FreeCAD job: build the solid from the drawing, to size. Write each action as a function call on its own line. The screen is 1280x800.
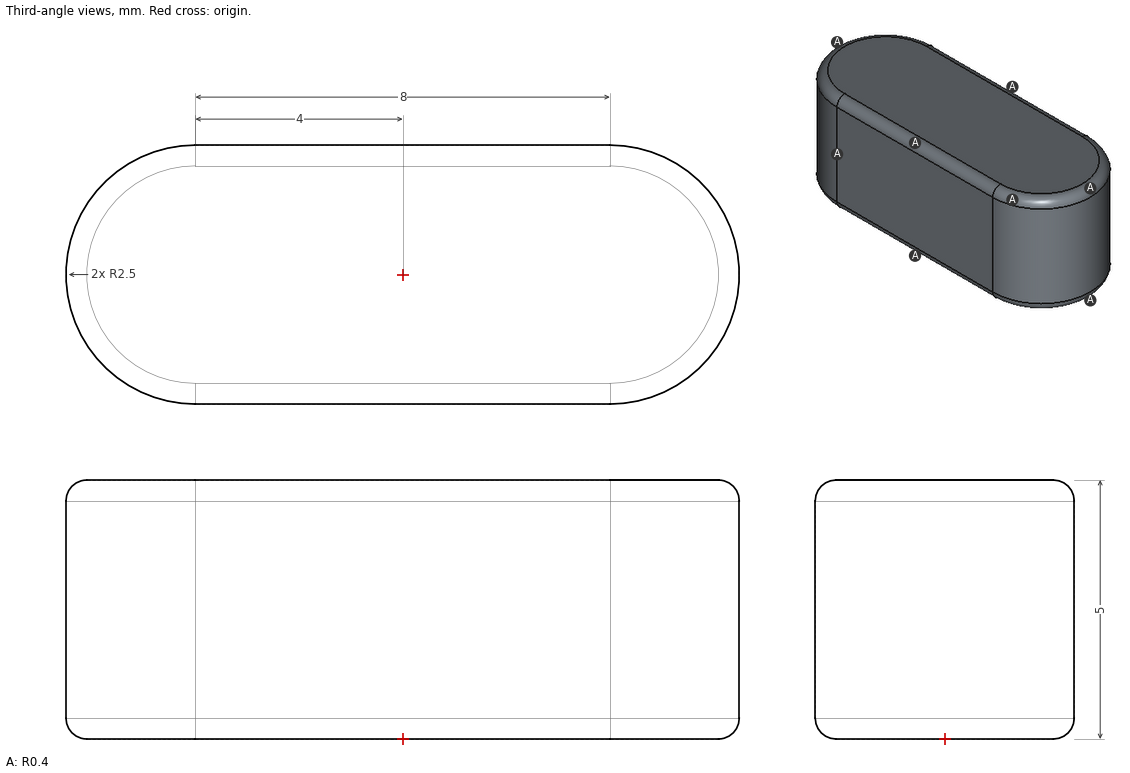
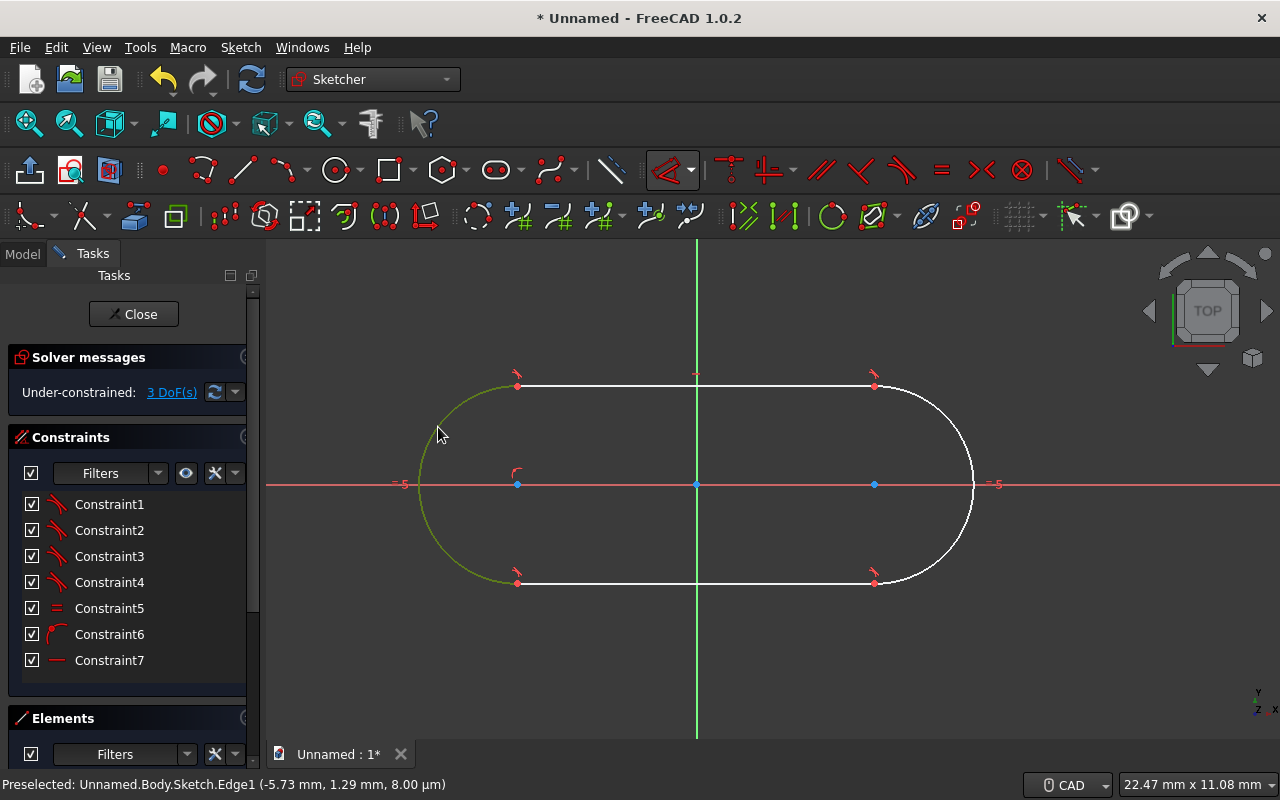
key(k)
key(r)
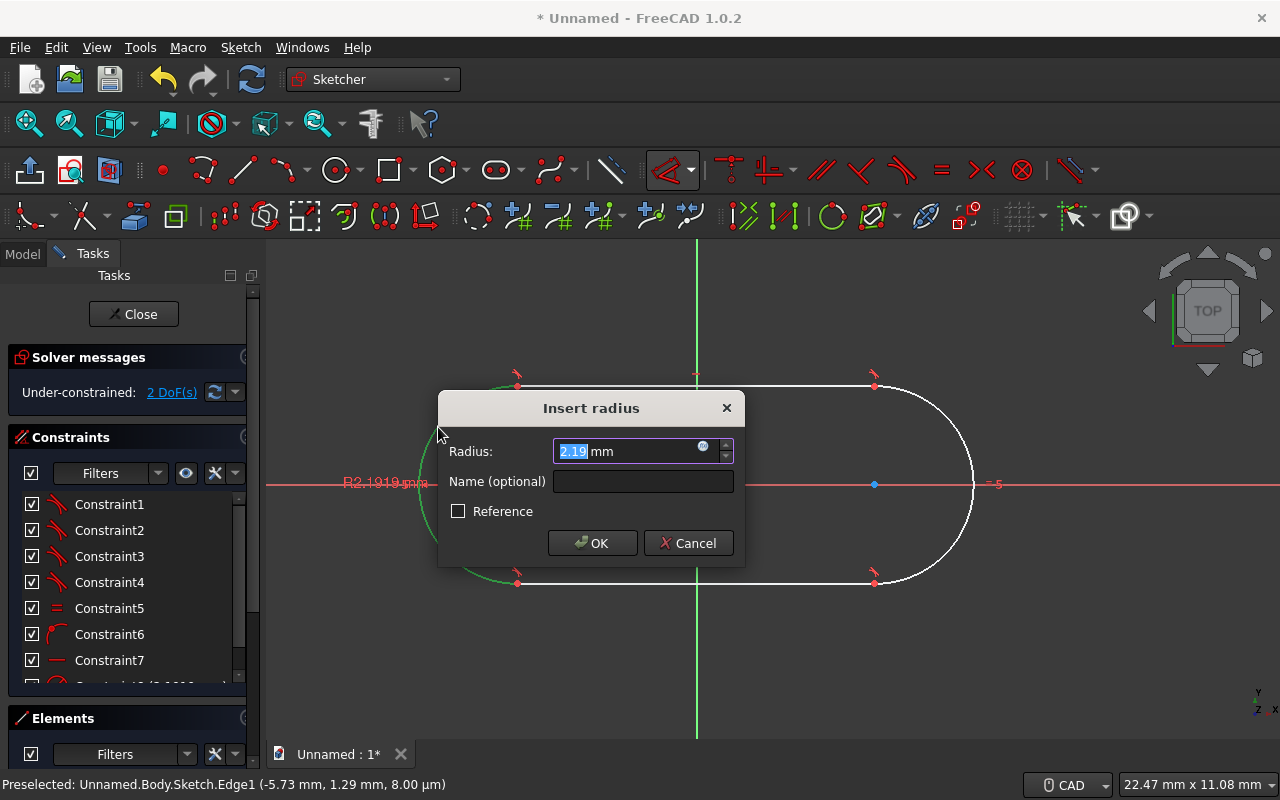
text(2.5)
key(Return)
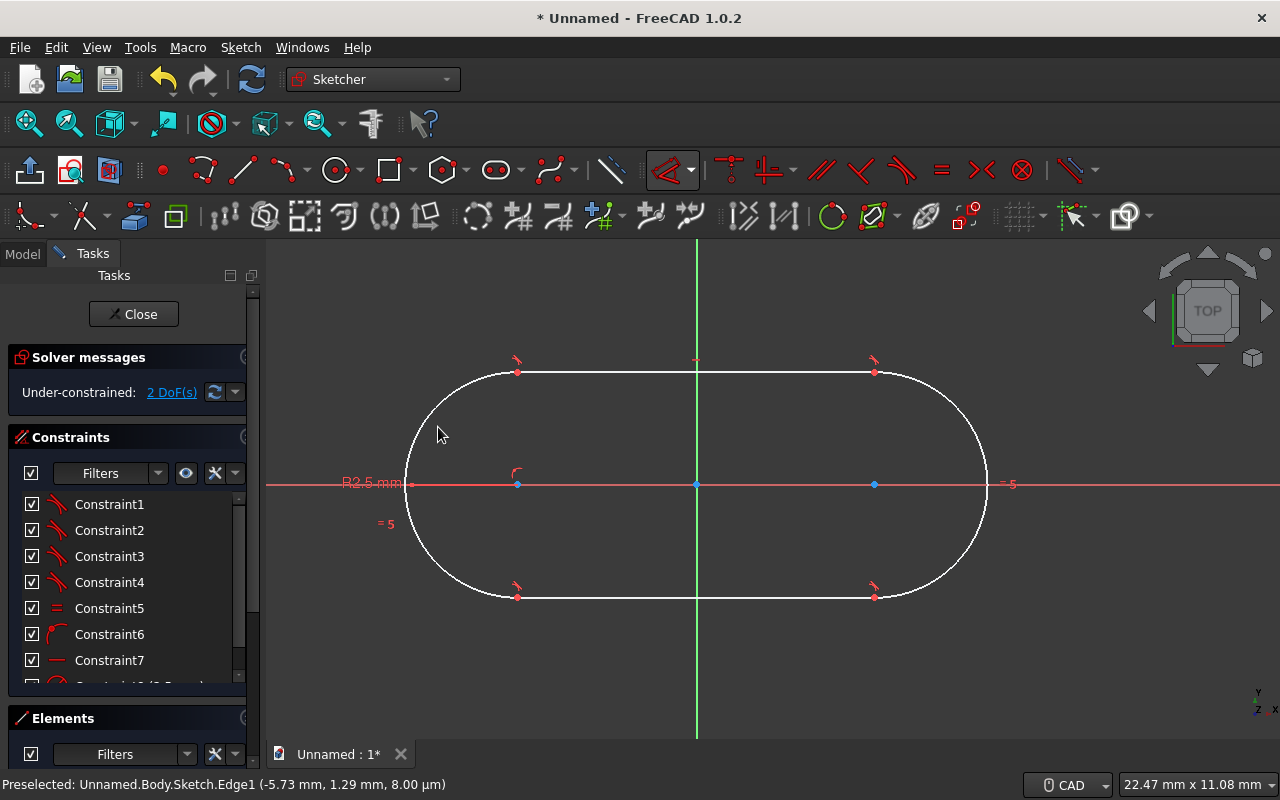
click(625, 372)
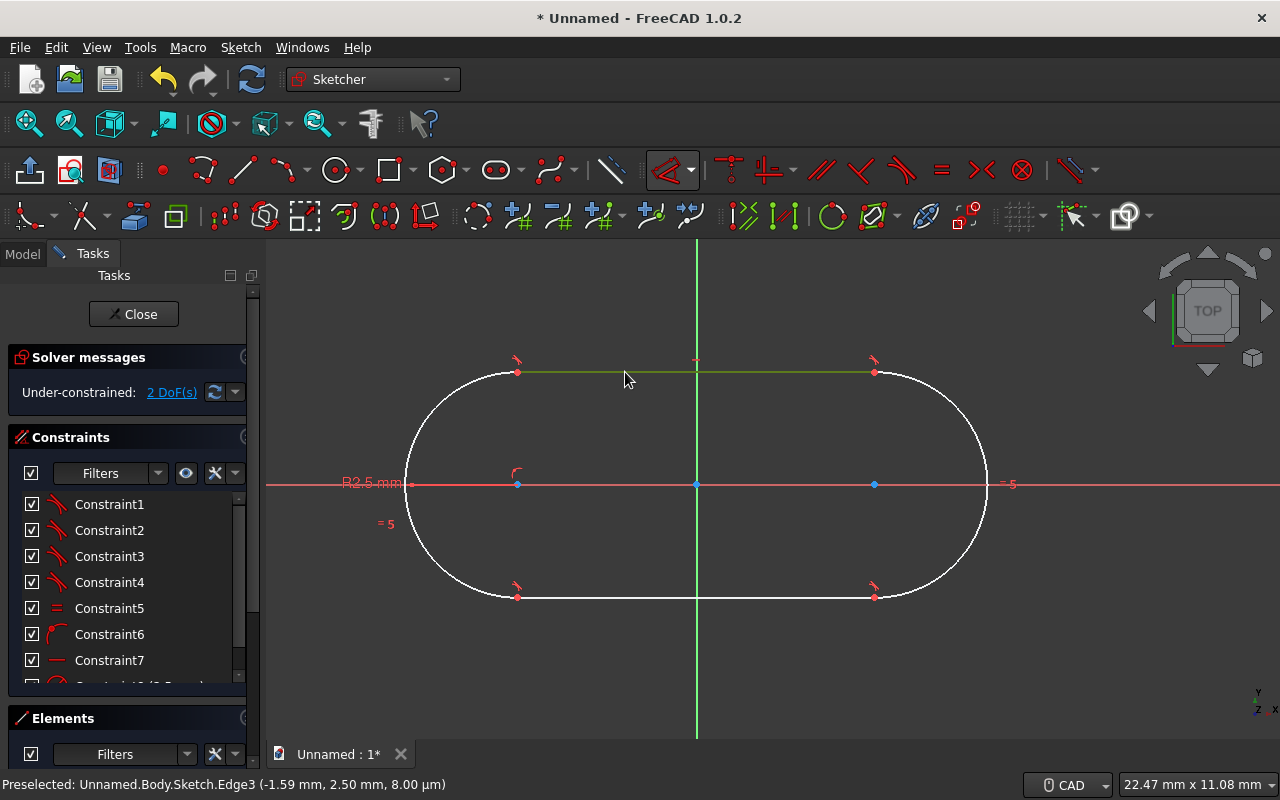
key(l)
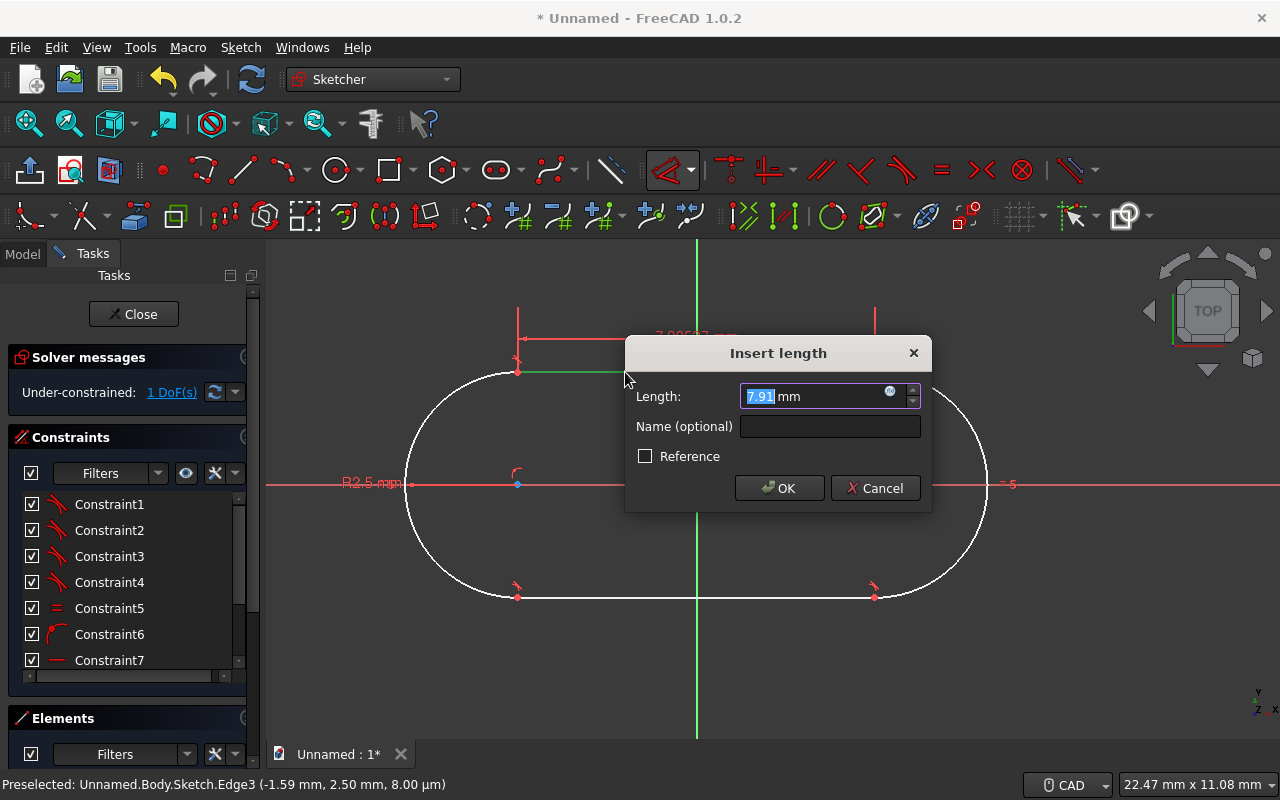
text(8)
key(Return)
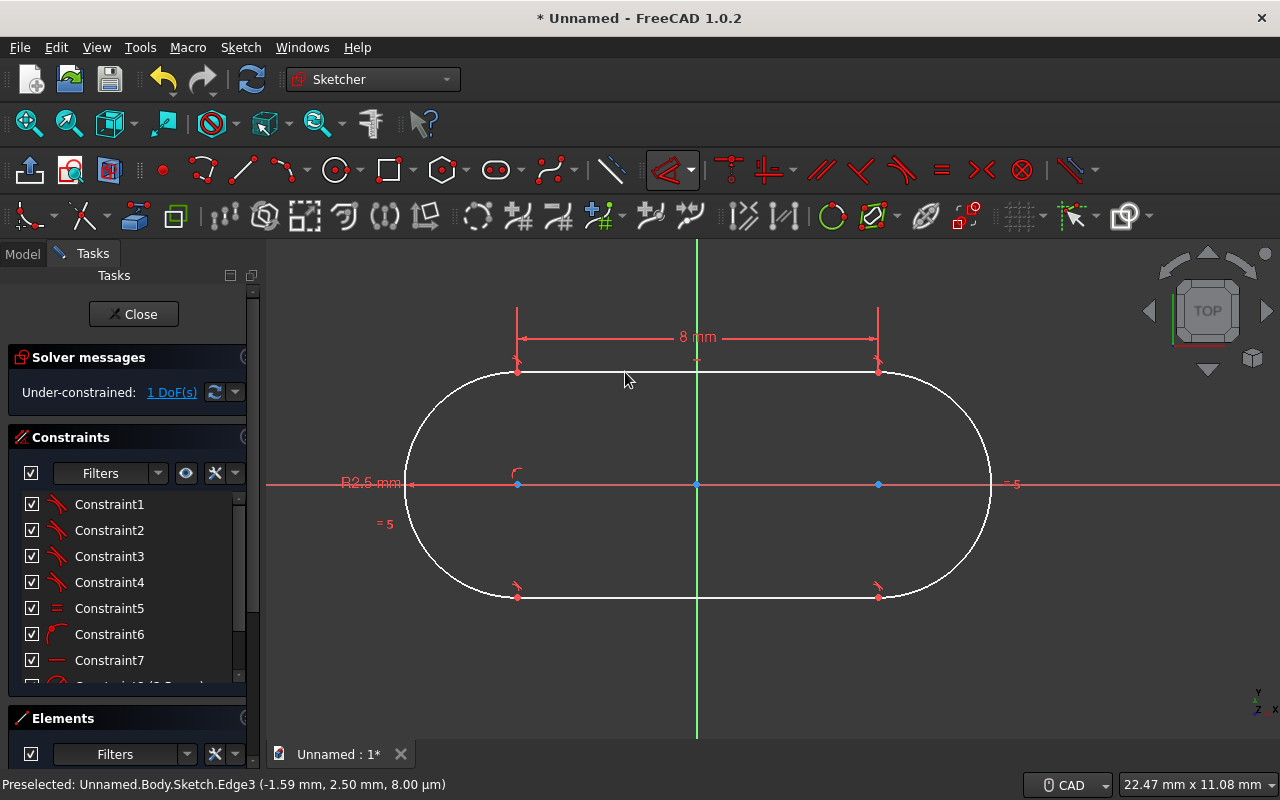
click(517, 372)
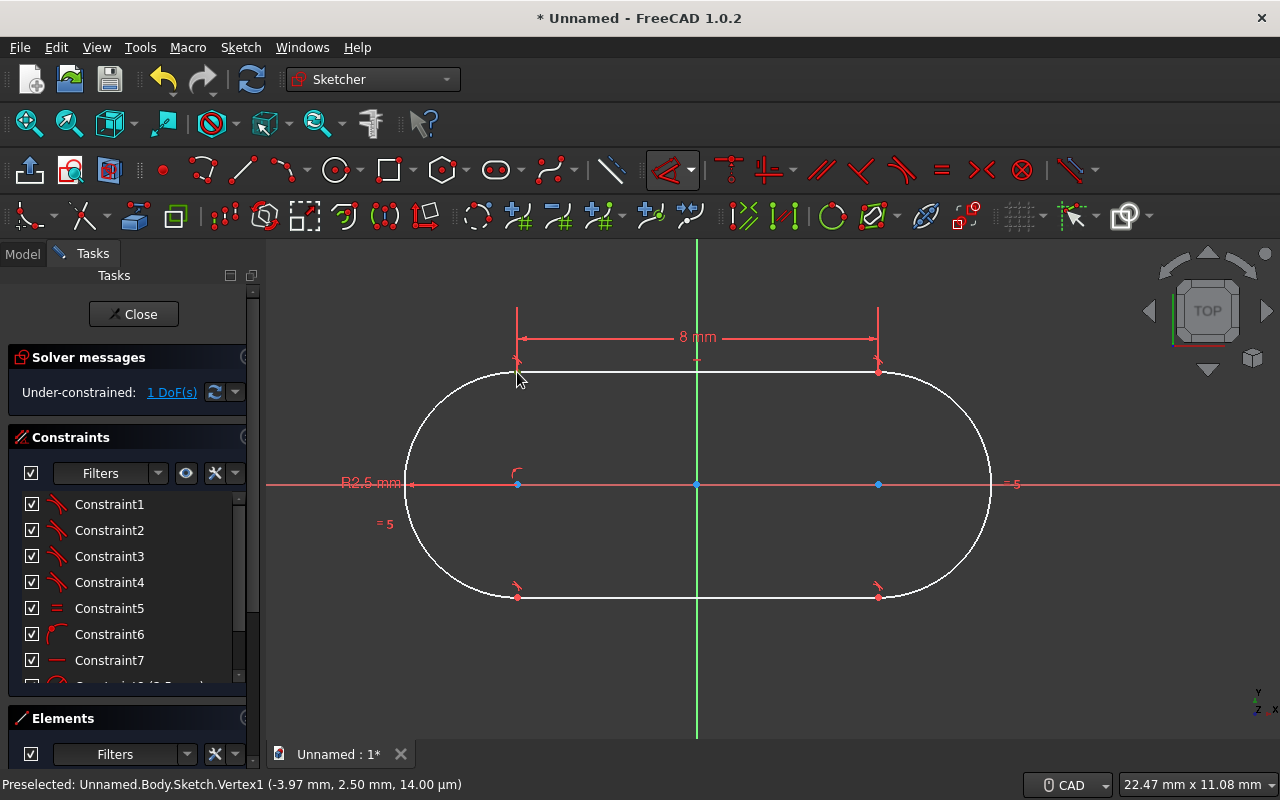
click(694, 170)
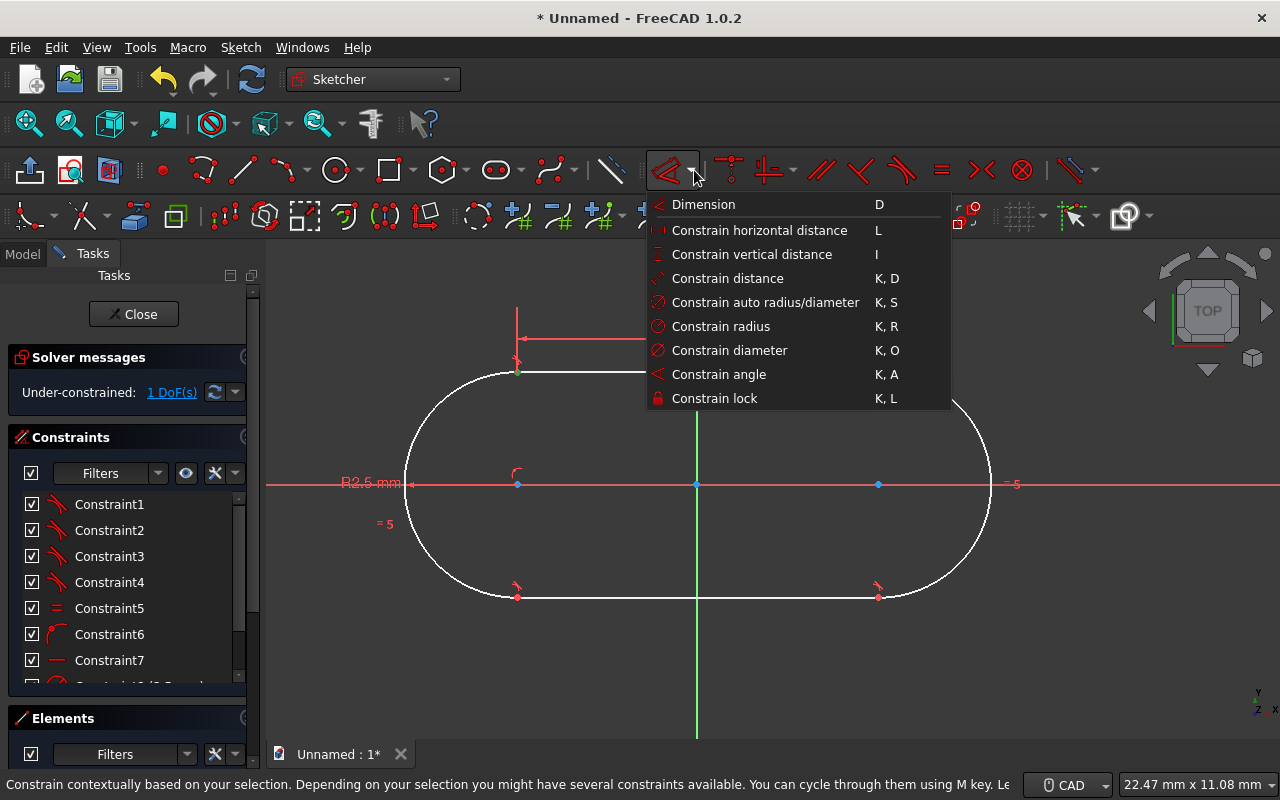
click(799, 230)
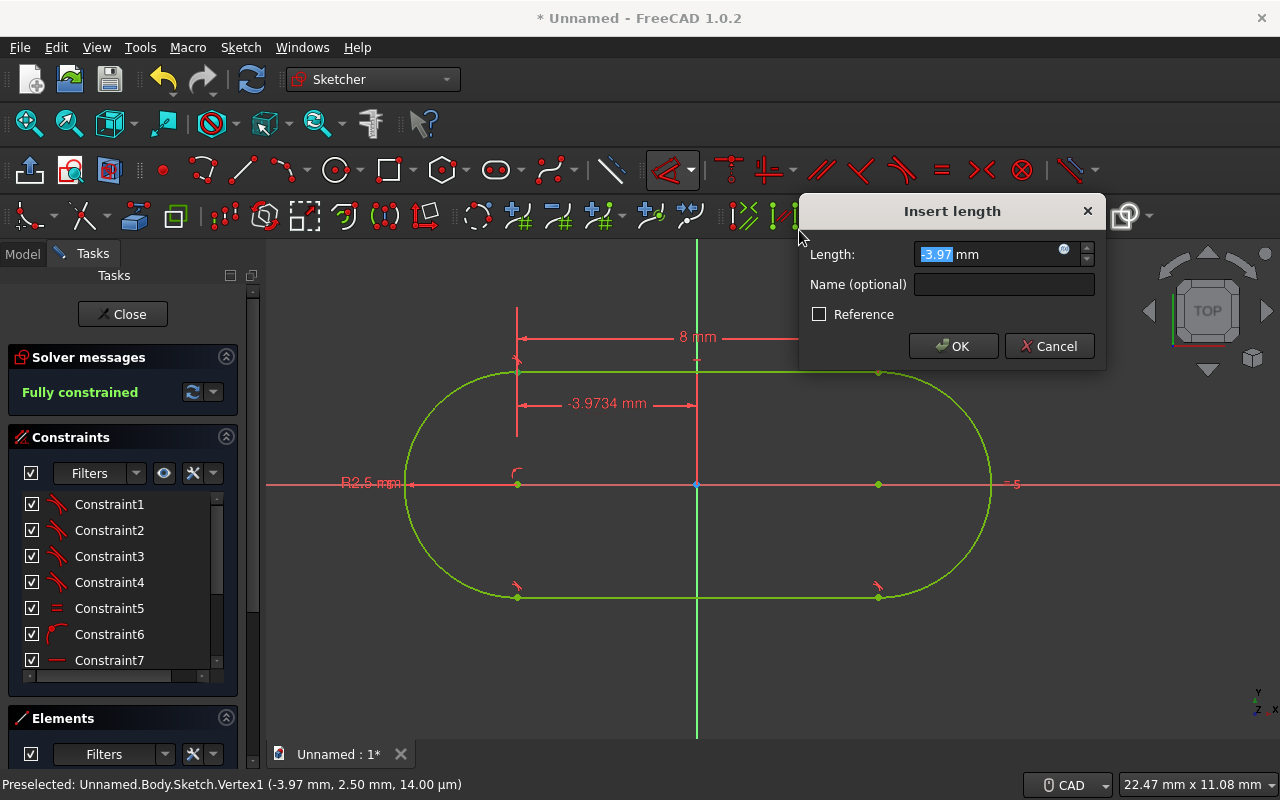
text(-4)
key(Return)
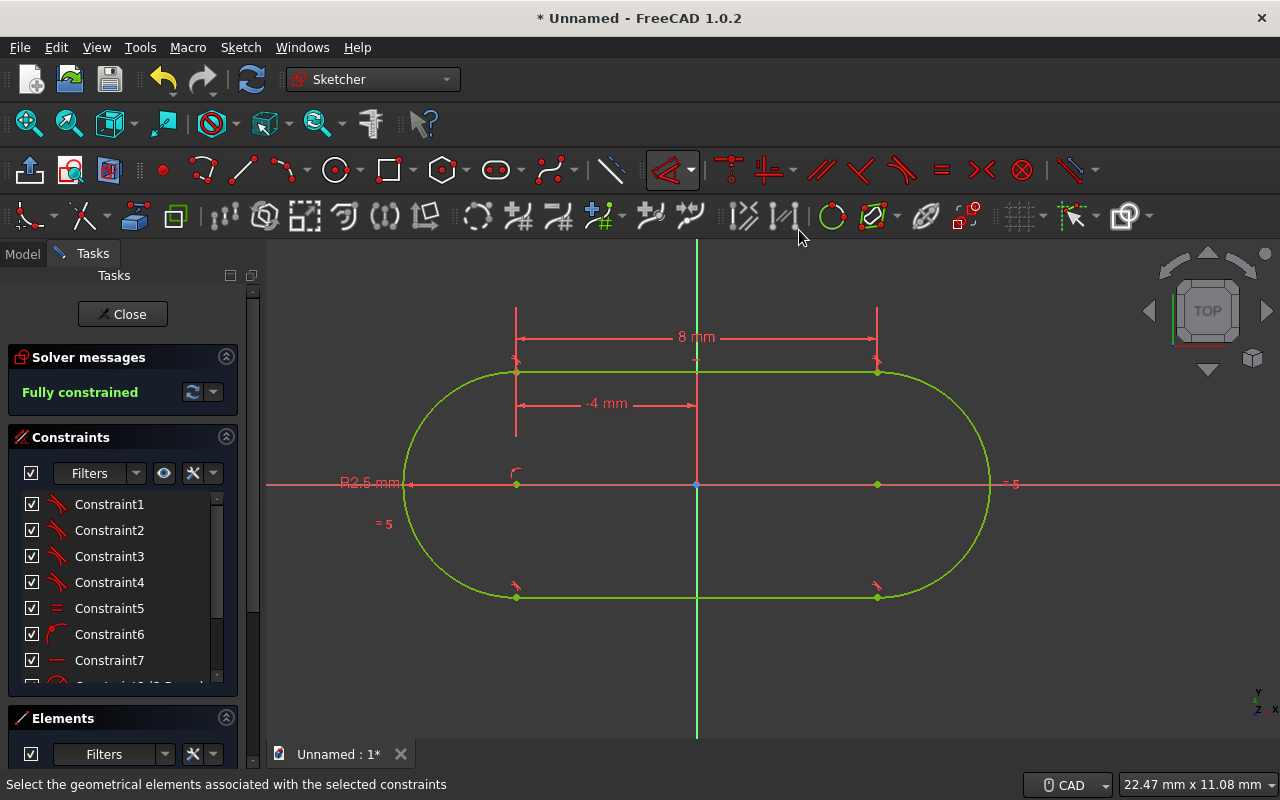
click(123, 314)